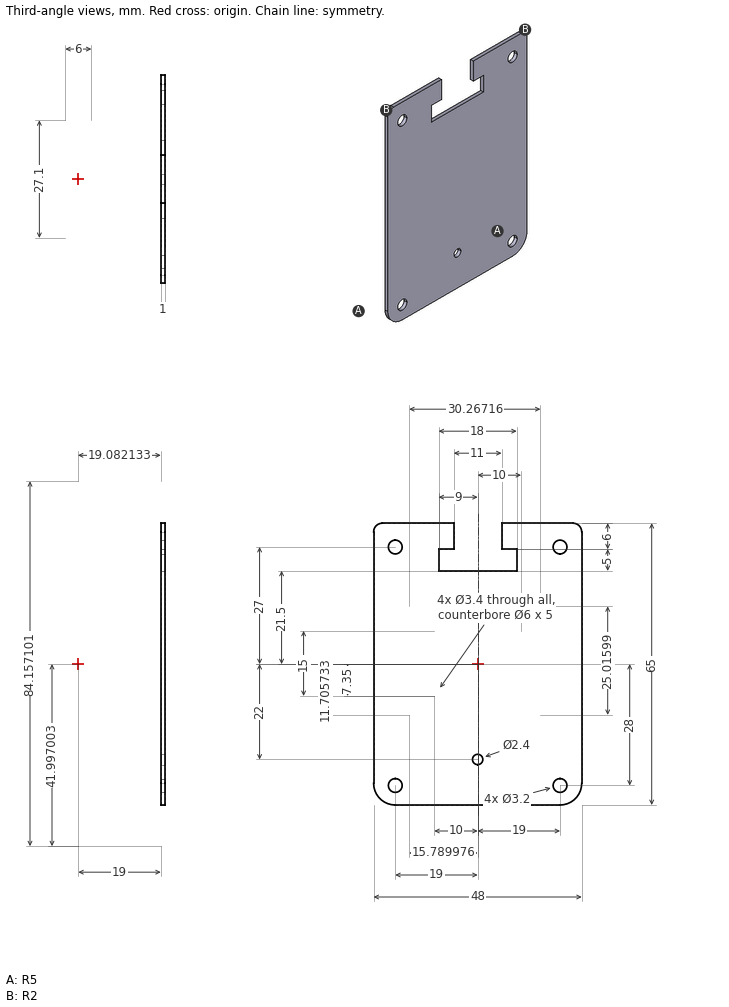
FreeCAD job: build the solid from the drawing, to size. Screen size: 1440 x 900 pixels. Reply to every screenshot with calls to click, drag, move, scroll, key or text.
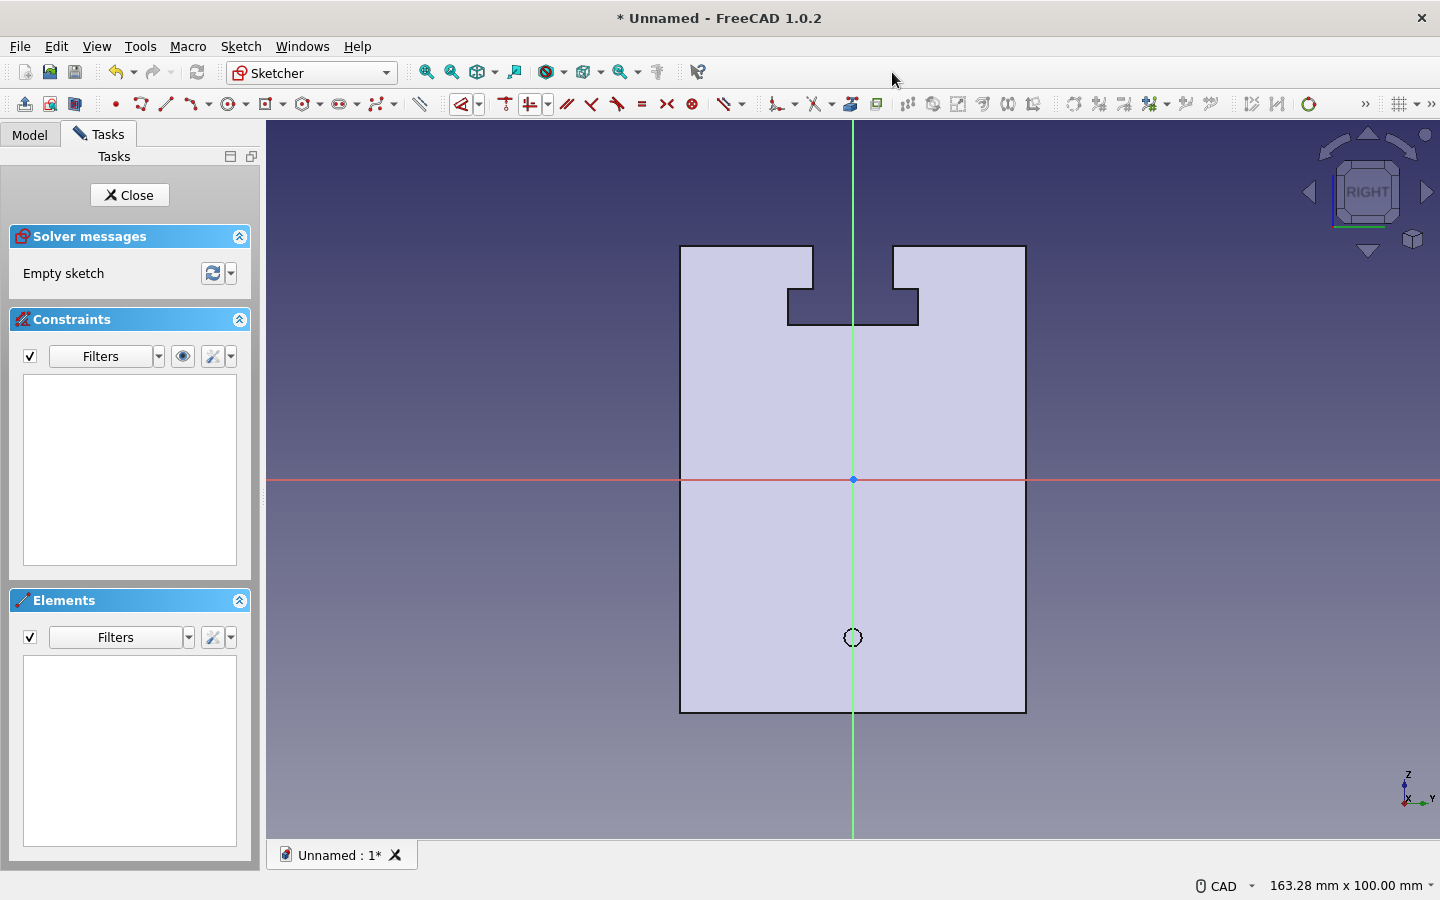
scroll(883, 478, up, 6)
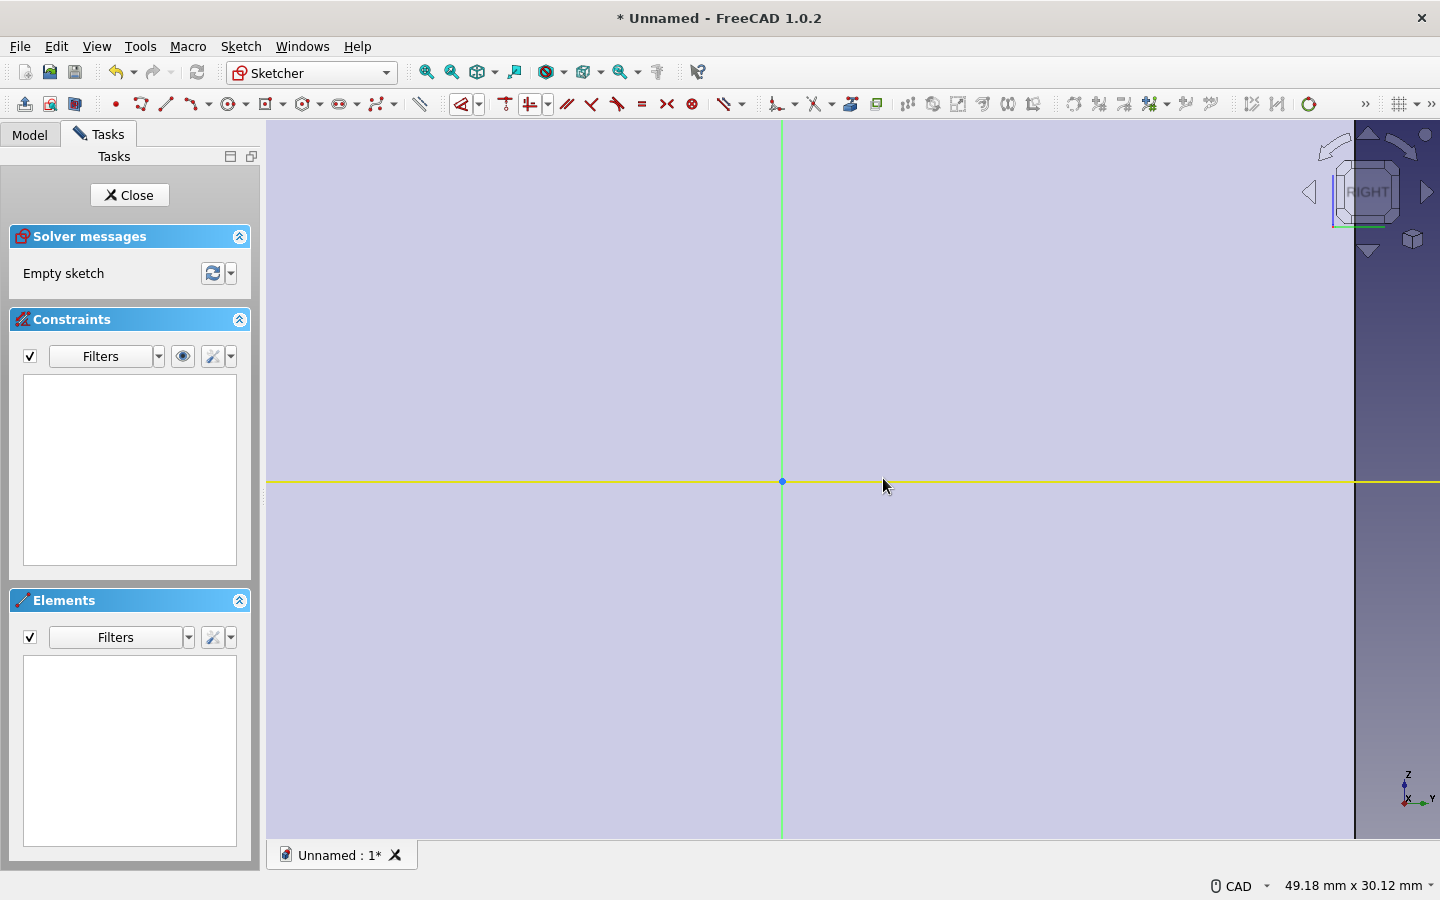
key(g)
key(c)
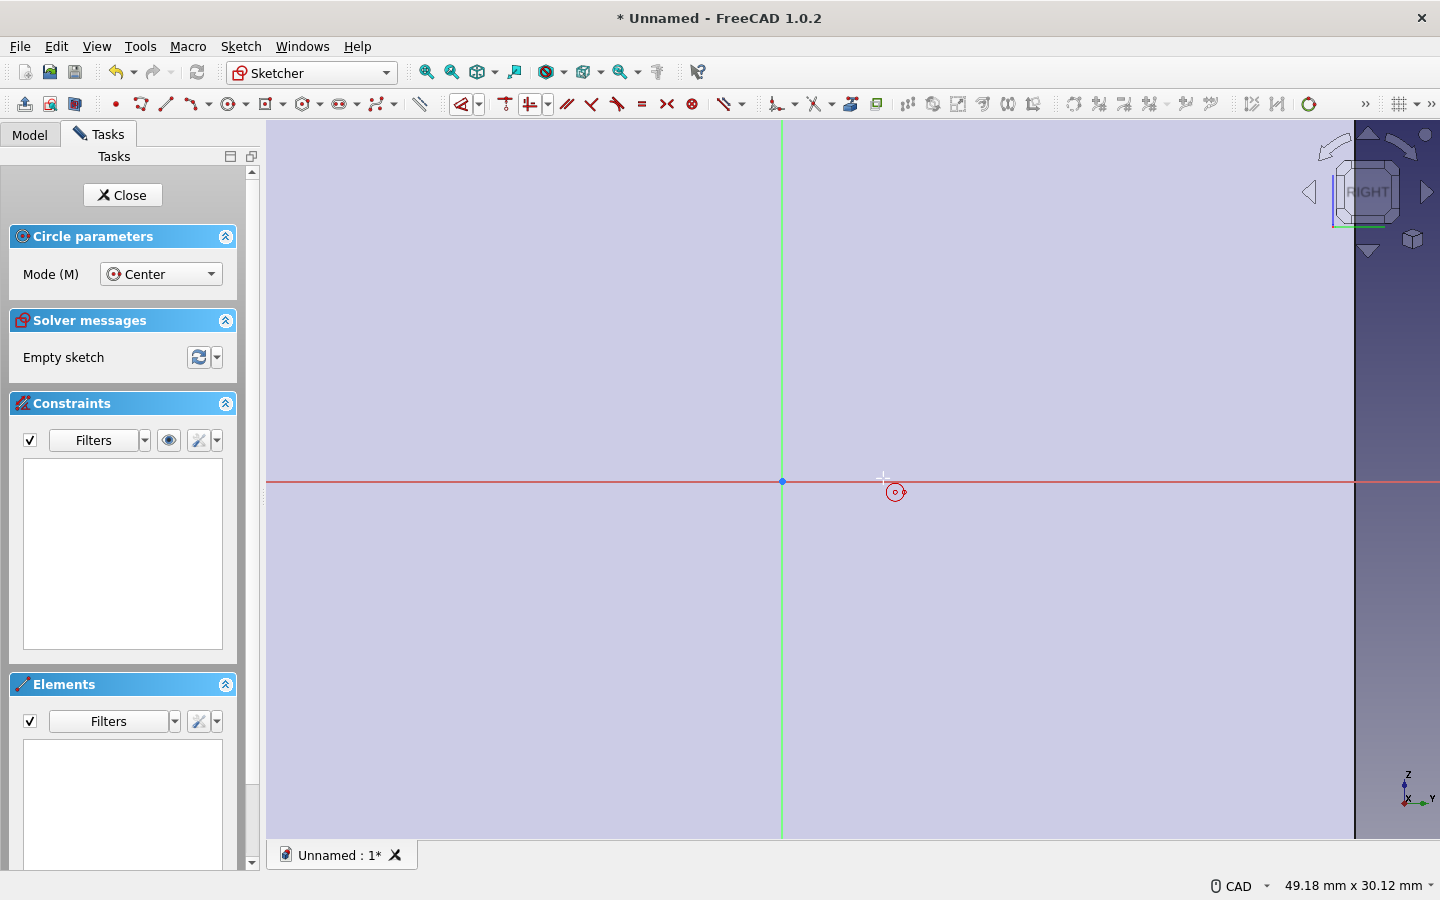
click(543, 657)
move(572, 629)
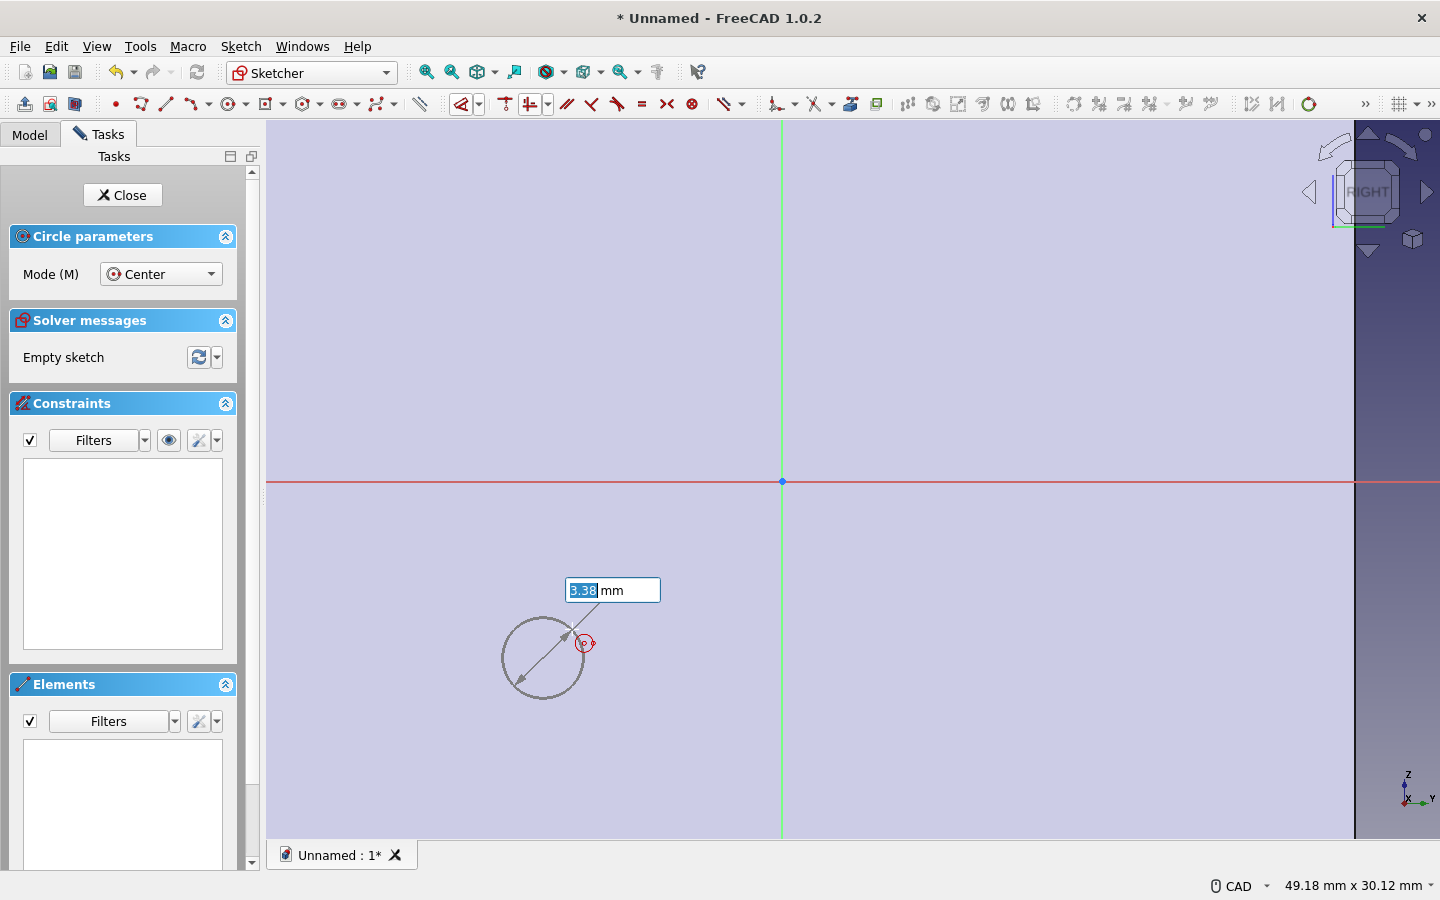
text(3.4)
key(Return)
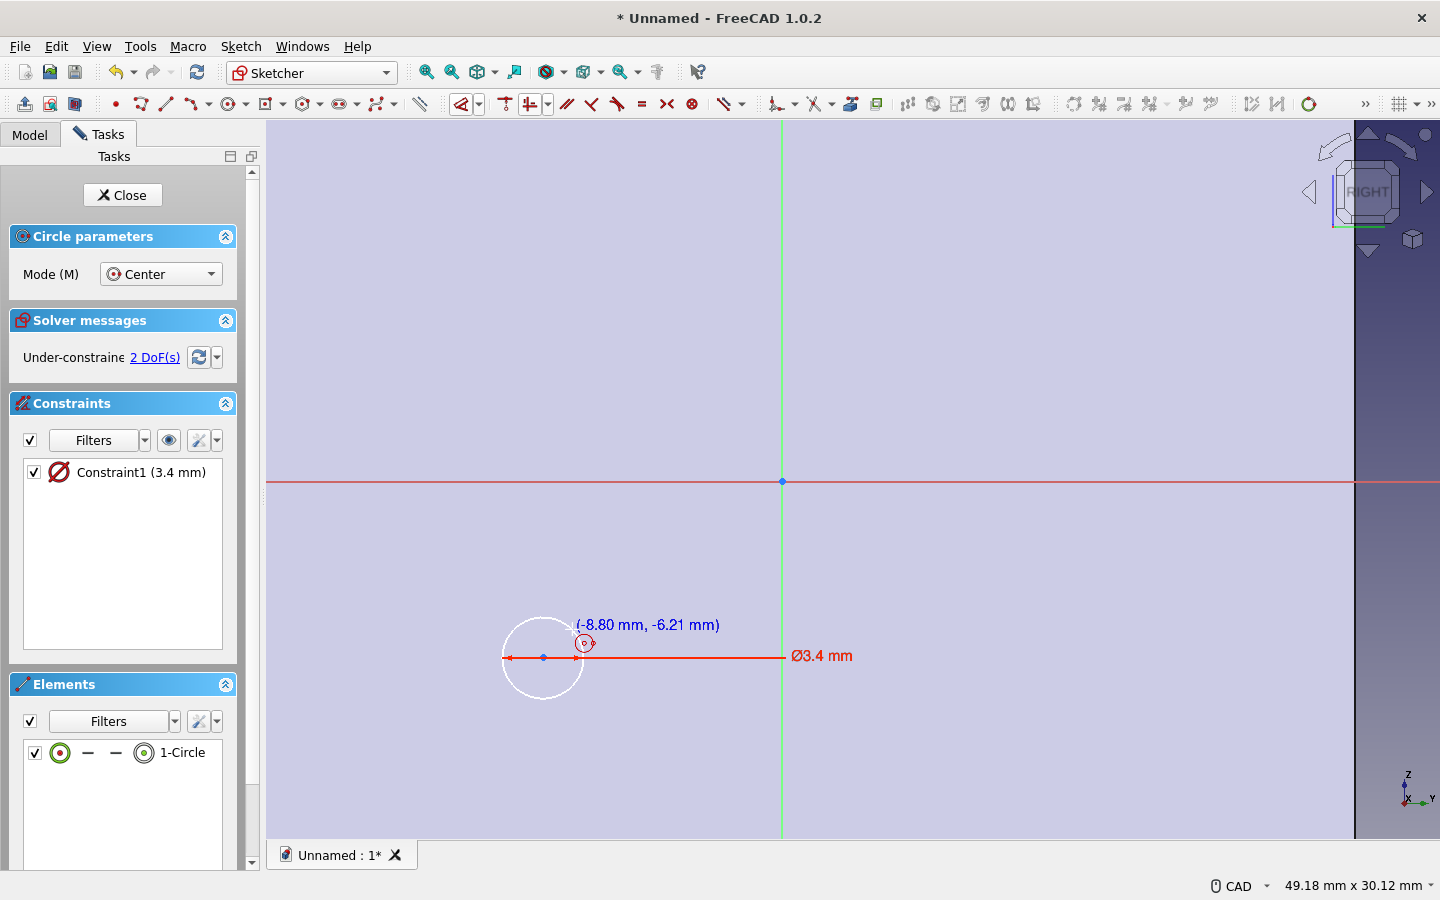
click(543, 299)
move(572, 271)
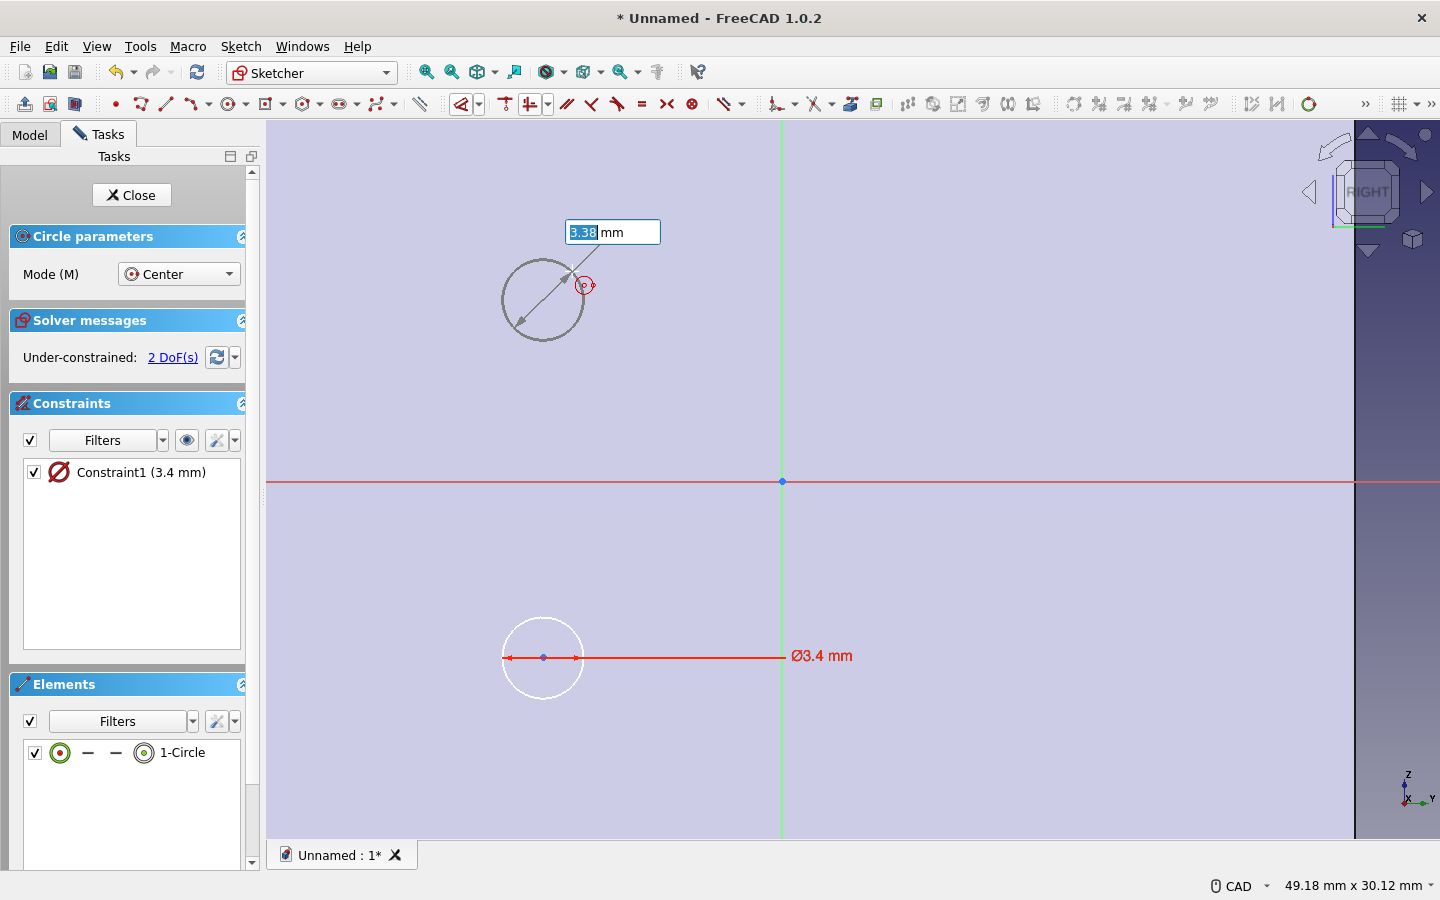
text(3.4)
key(Return)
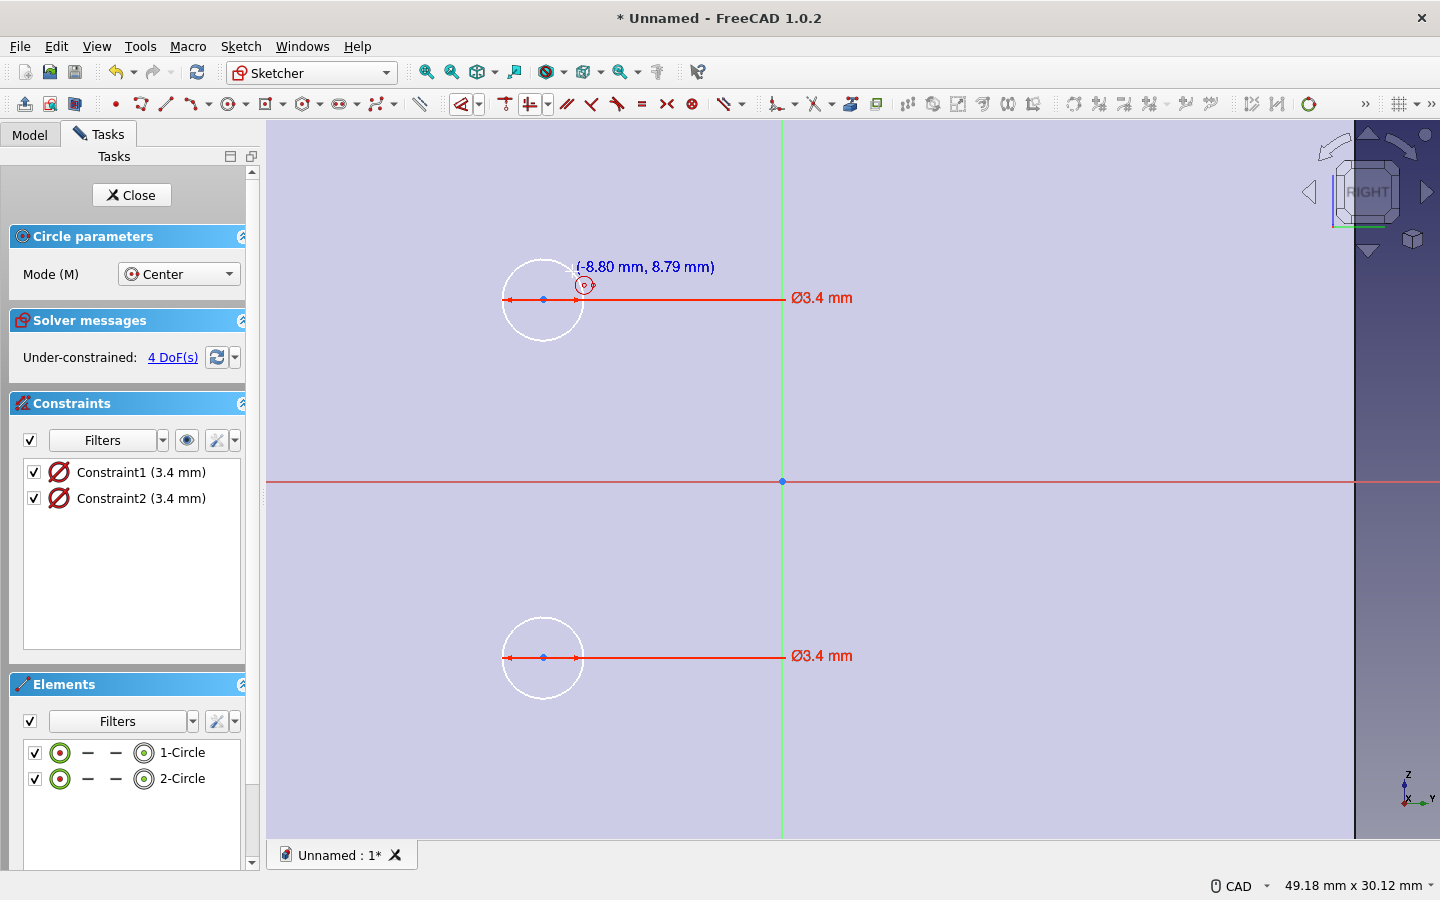
click(1021, 299)
move(1050, 271)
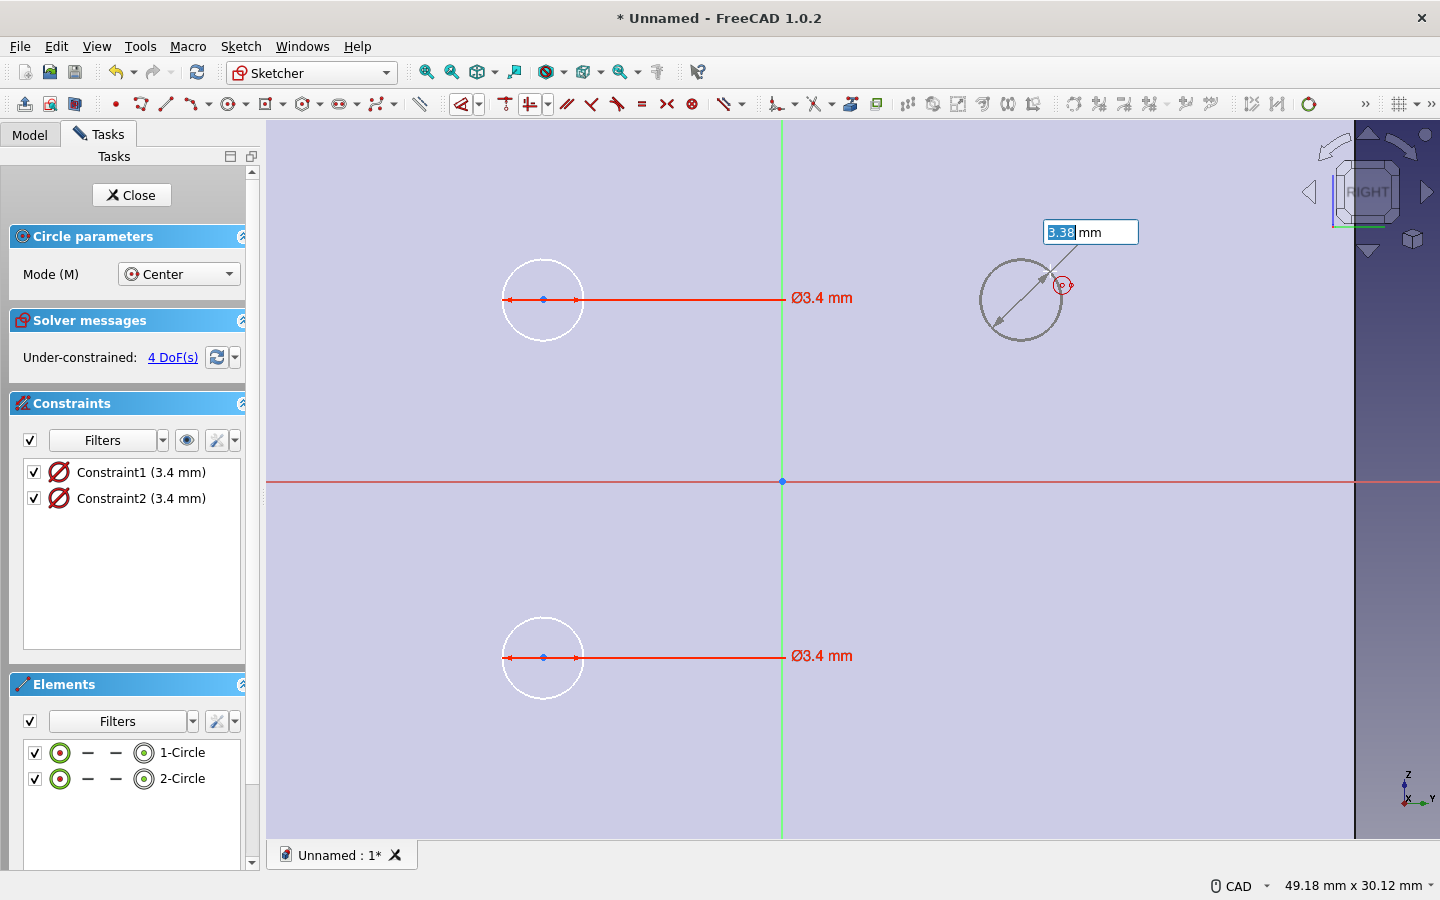
text(3.4)
key(Return)